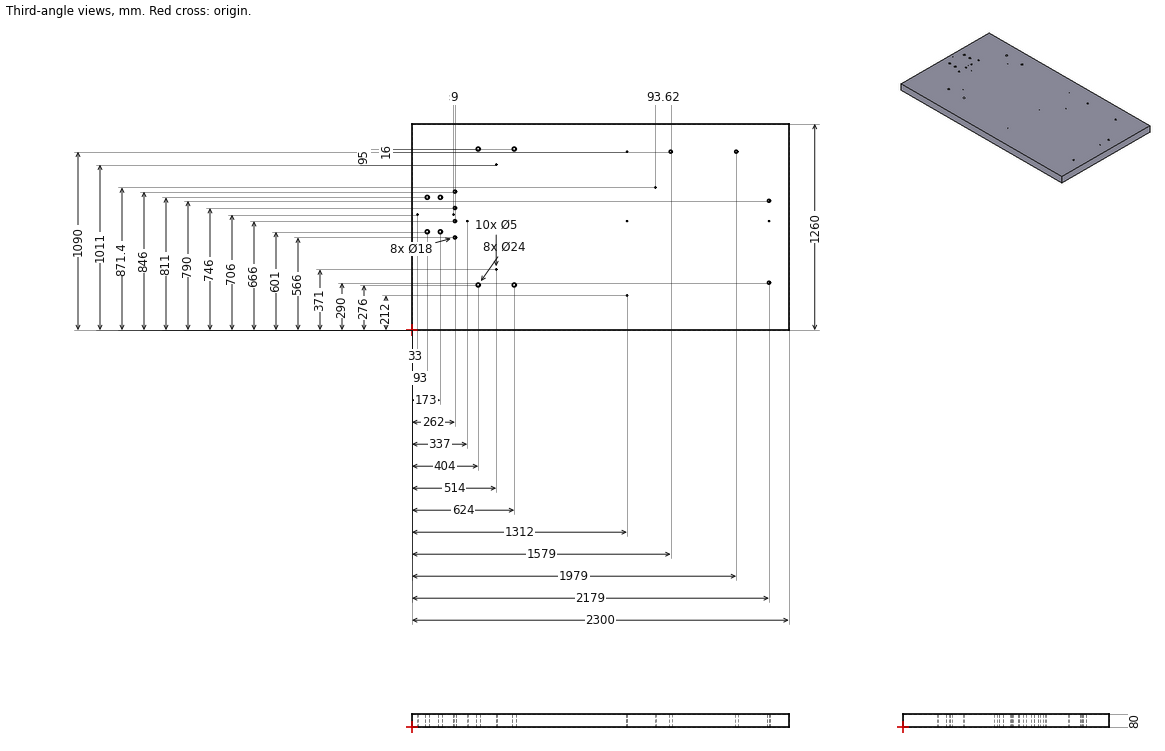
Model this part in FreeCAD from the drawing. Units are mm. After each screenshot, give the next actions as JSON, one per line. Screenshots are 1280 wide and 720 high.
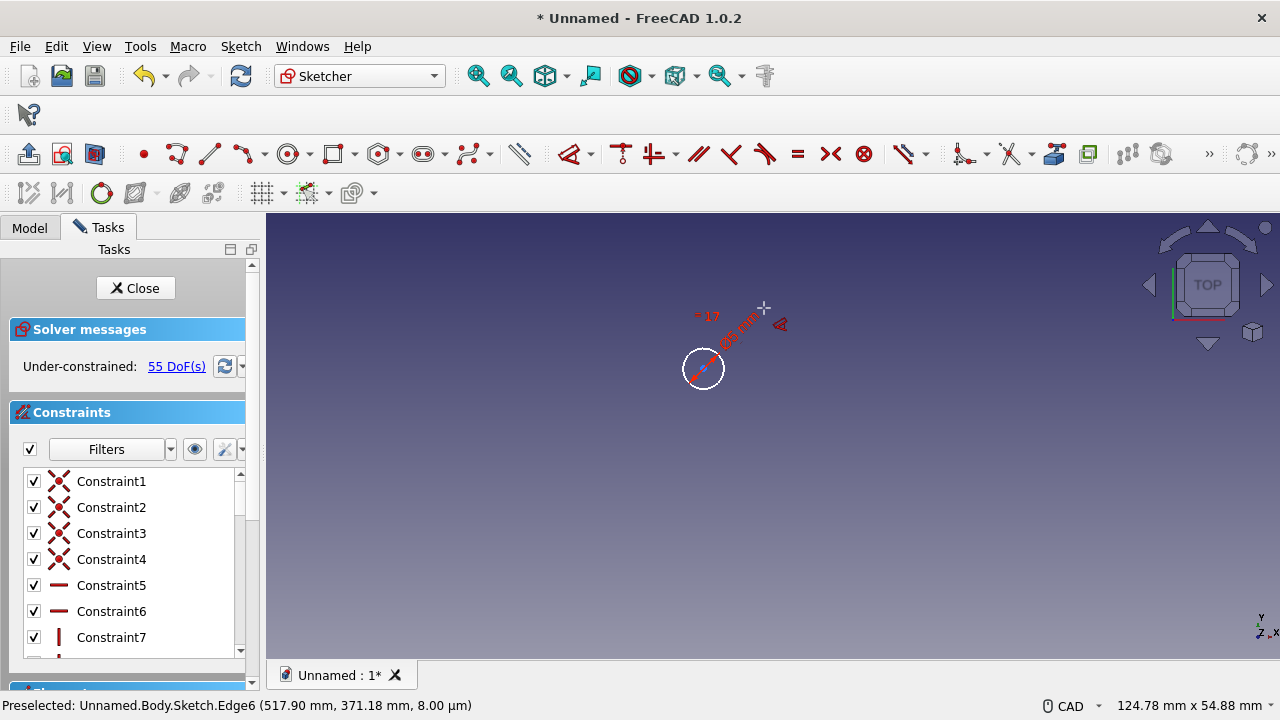
{"action": "scroll", "coordinate": [559, 498], "scroll_direction": "down", "scroll_amount": 18}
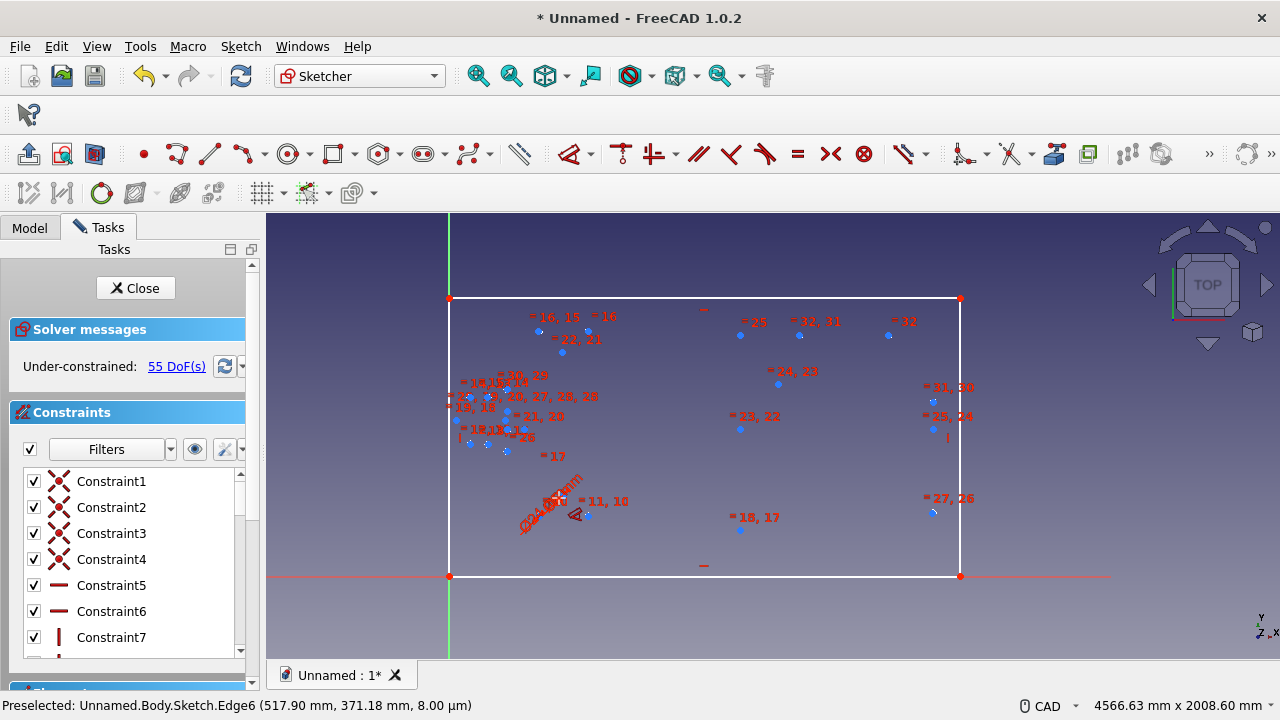
{"action": "scroll", "coordinate": [509, 450], "scroll_direction": "up", "scroll_amount": 12}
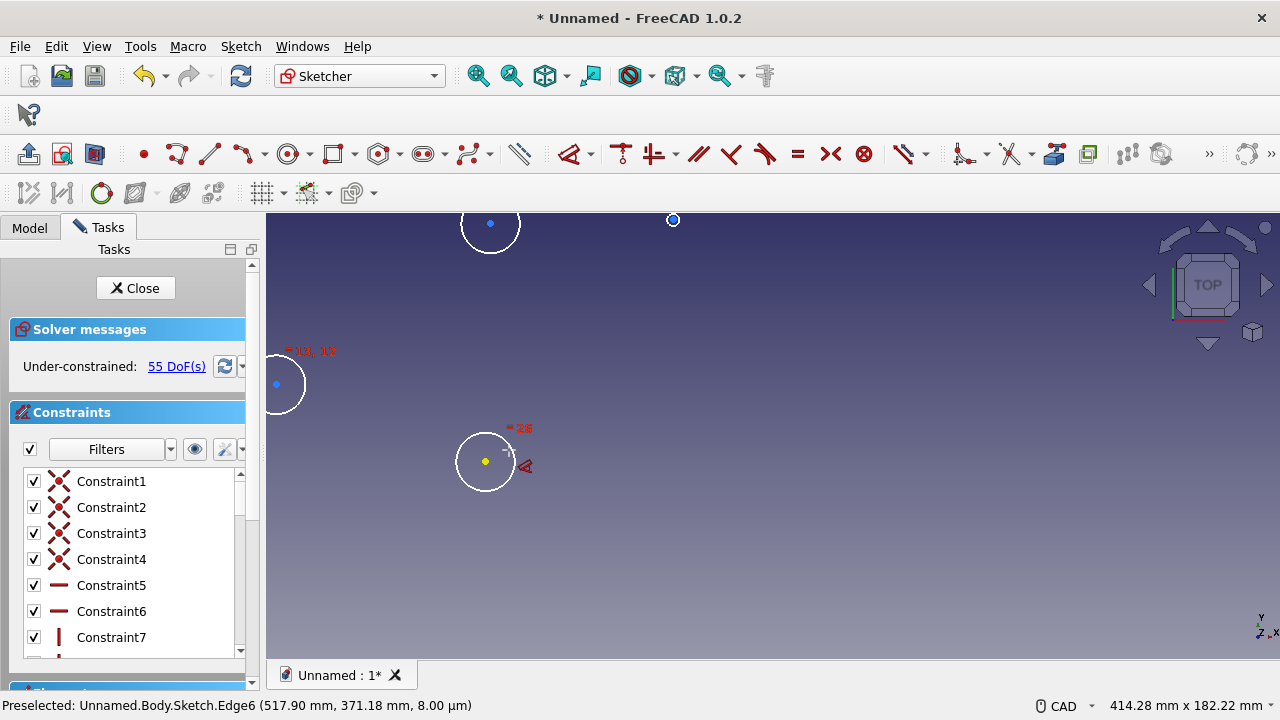
{"action": "left_click", "coordinate": [506, 441]}
{"action": "left_click", "coordinate": [528, 418]}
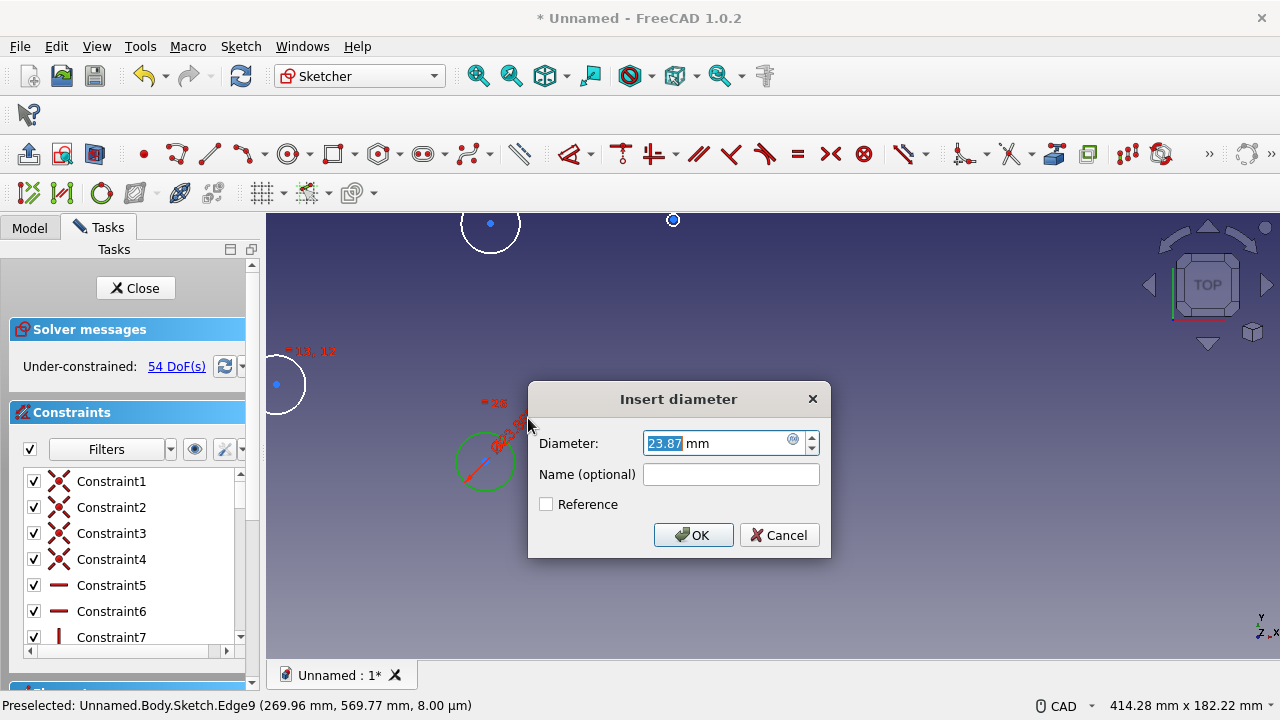
{"action": "type", "text": "18"}
{"action": "key", "text": "Return"}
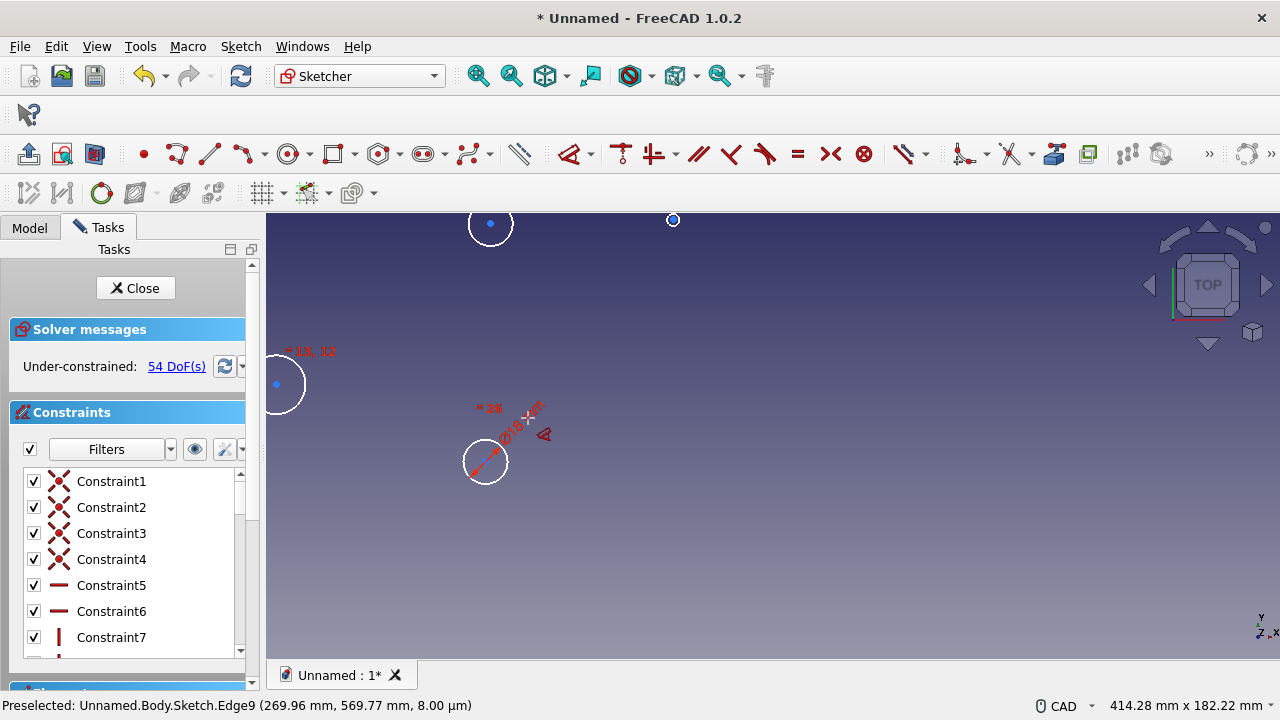
{"action": "scroll", "coordinate": [509, 450], "scroll_direction": "down", "scroll_amount": 12}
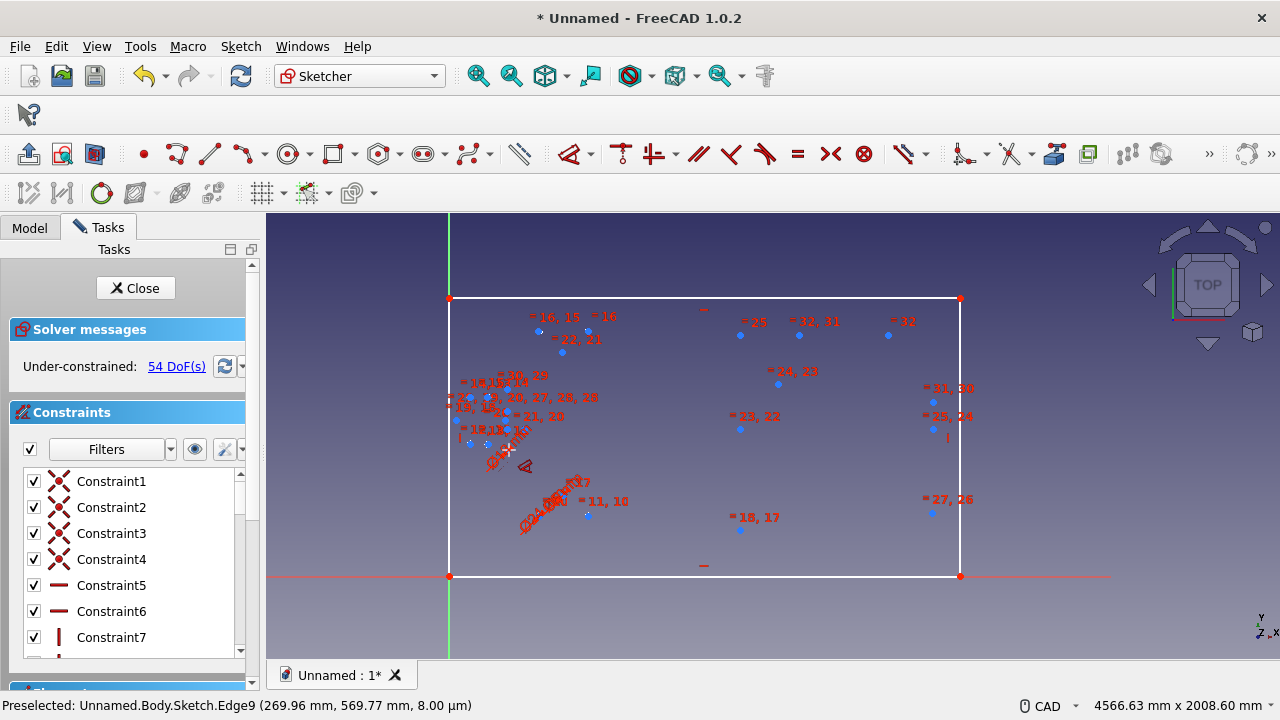
{"action": "scroll", "coordinate": [470, 444], "scroll_direction": "up", "scroll_amount": 4}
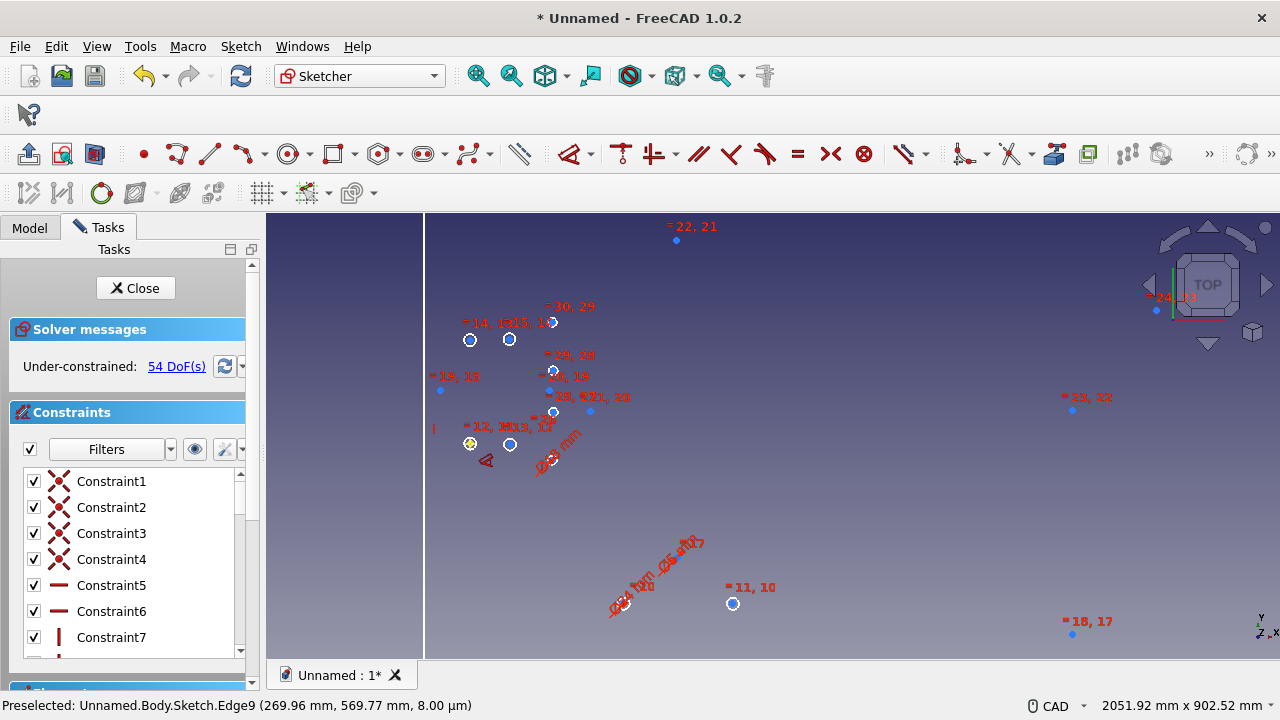
{"action": "left_click", "coordinate": [470, 444]}
{"action": "left_click", "coordinate": [447, 410]}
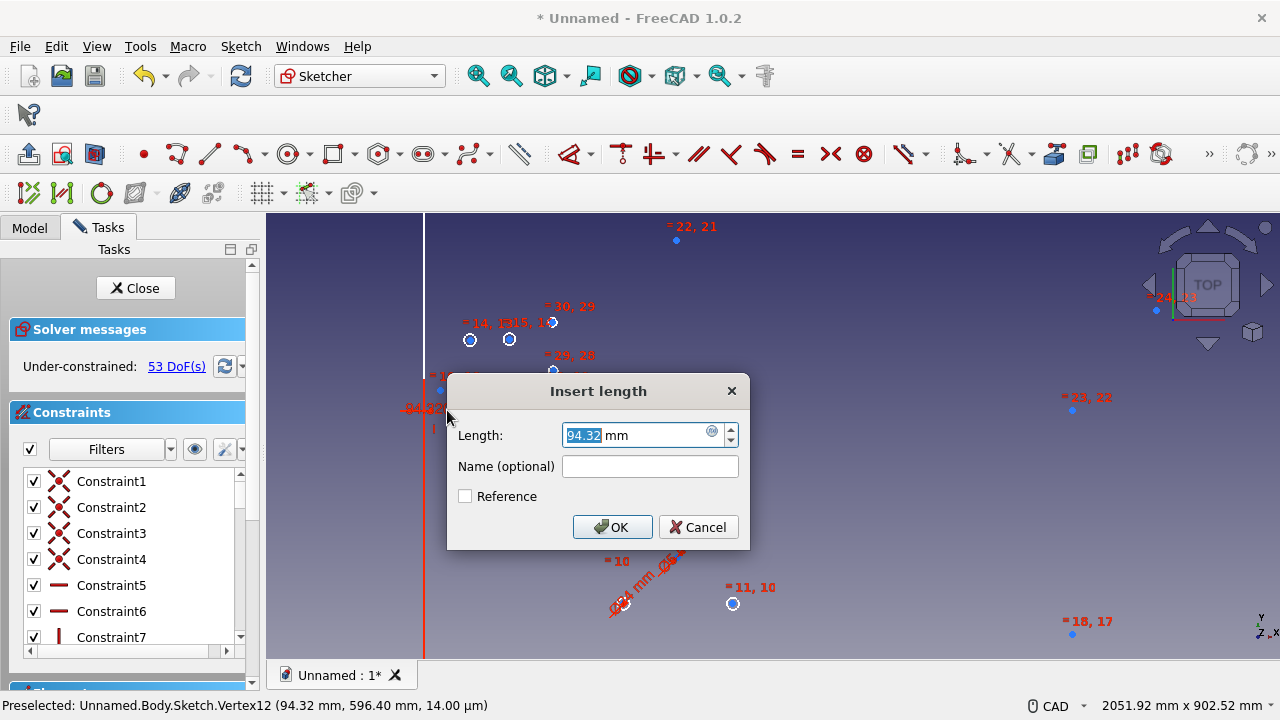
{"action": "type", "text": "93"}
{"action": "key", "text": "Return"}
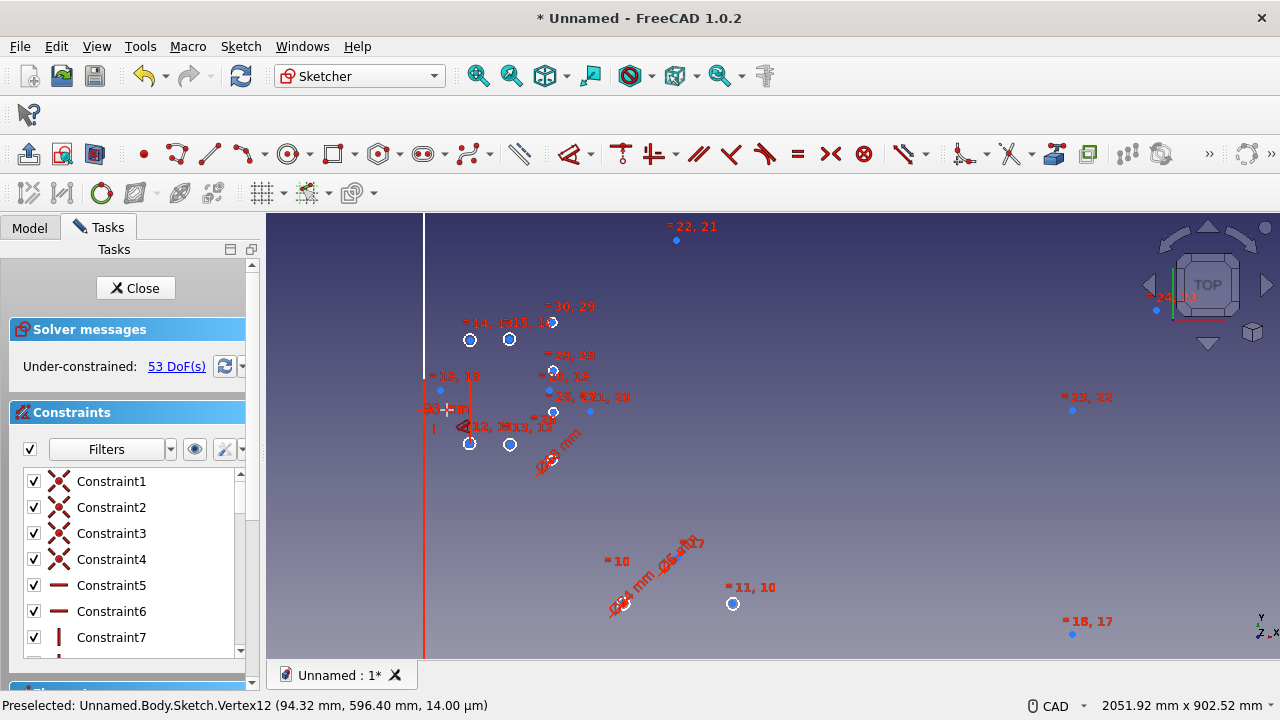
{"action": "scroll", "coordinate": [440, 390], "scroll_direction": "up", "scroll_amount": 5}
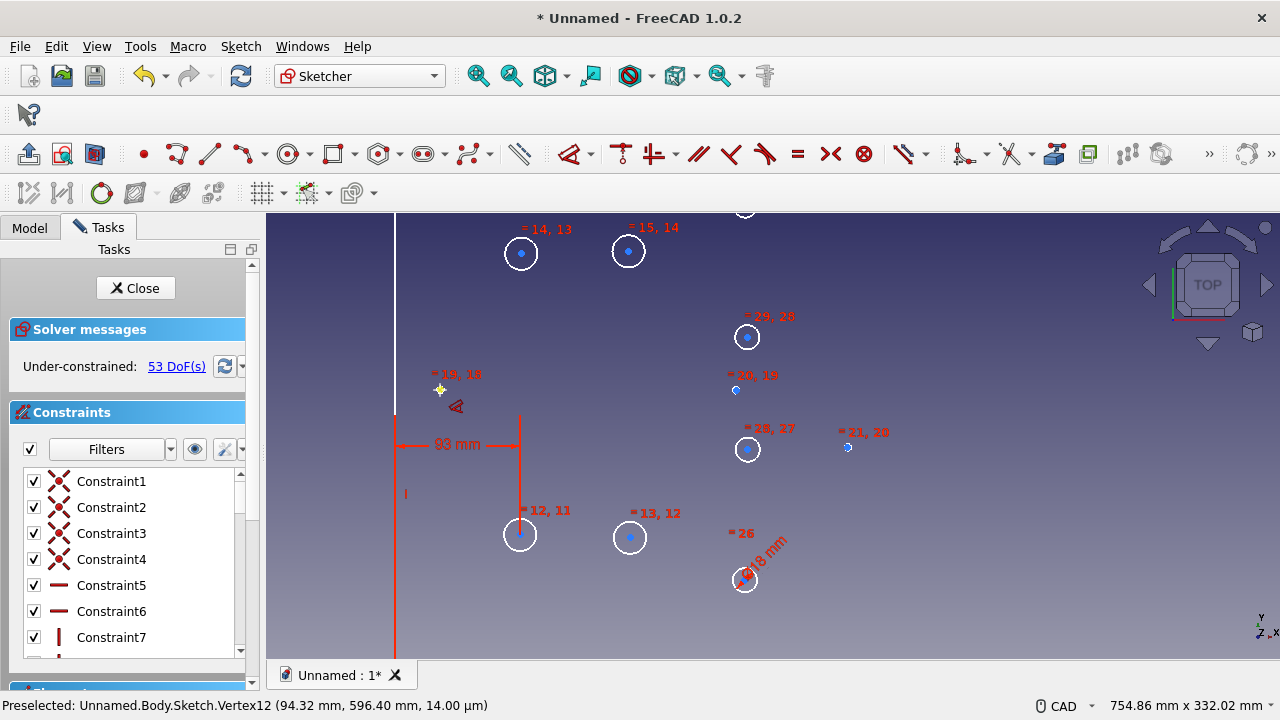
{"action": "left_click", "coordinate": [441, 390]}
{"action": "left_click", "coordinate": [418, 356]}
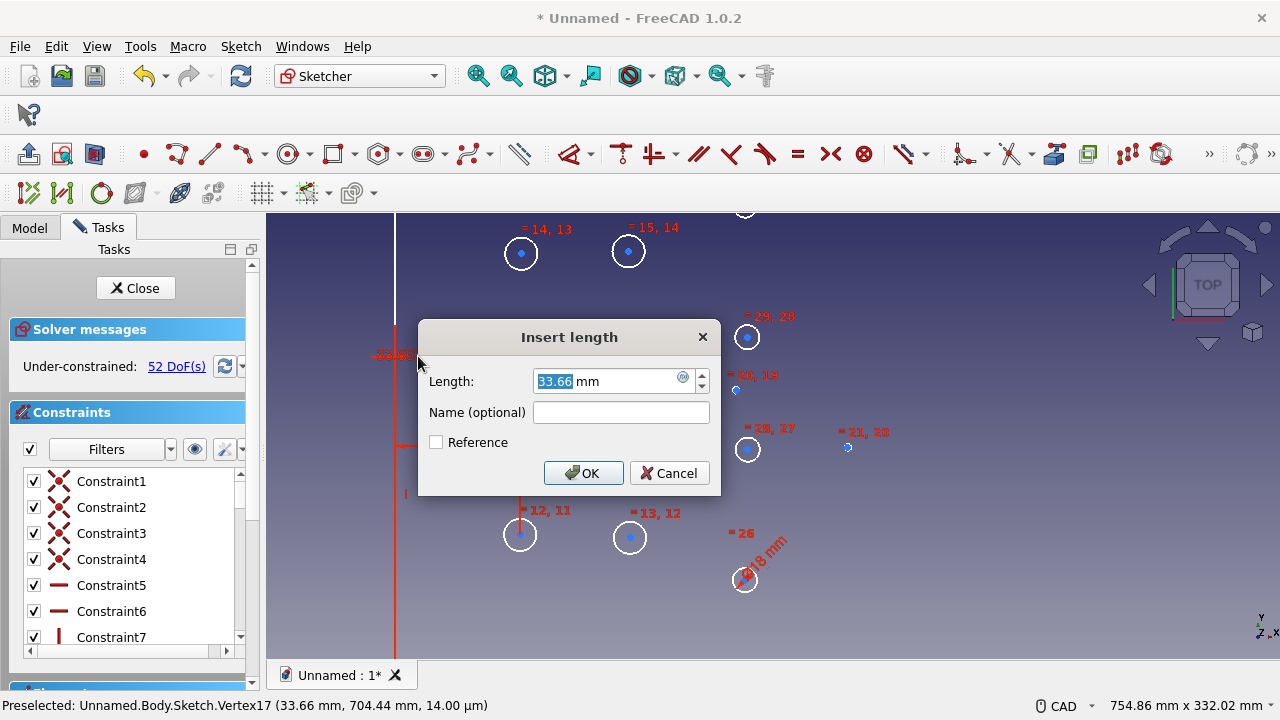
{"action": "type", "text": "33"}
{"action": "key", "text": "Return"}